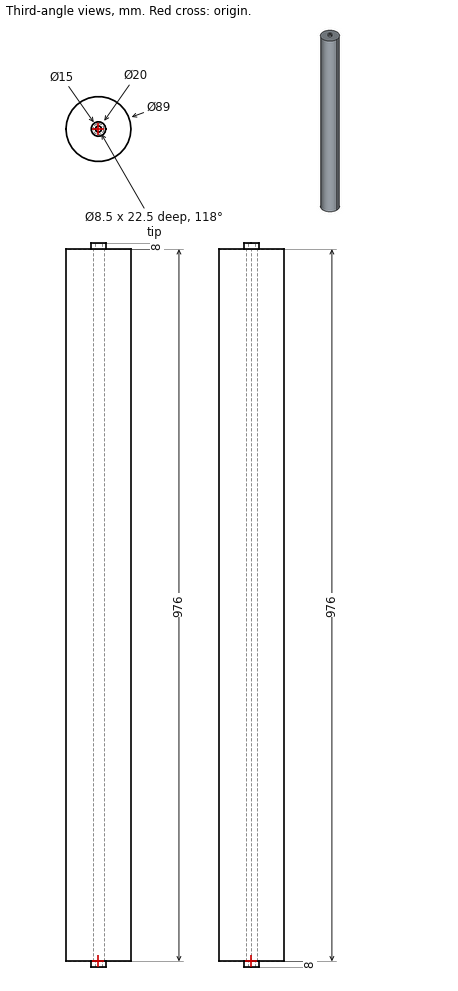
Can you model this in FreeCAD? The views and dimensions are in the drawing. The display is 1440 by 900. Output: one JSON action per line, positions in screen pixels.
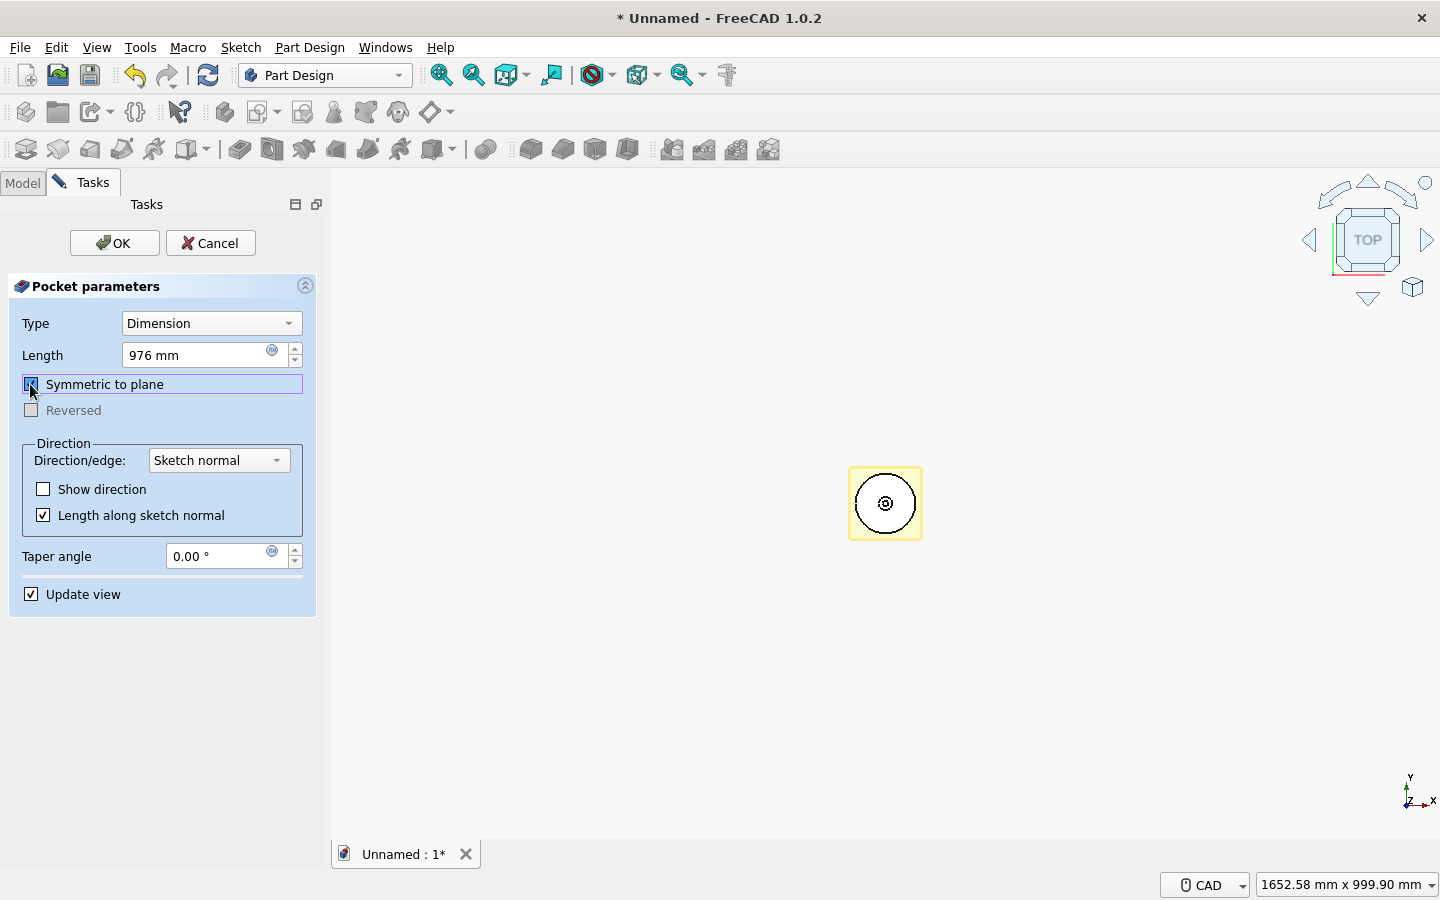
{"action": "left_click", "coordinate": [115, 243]}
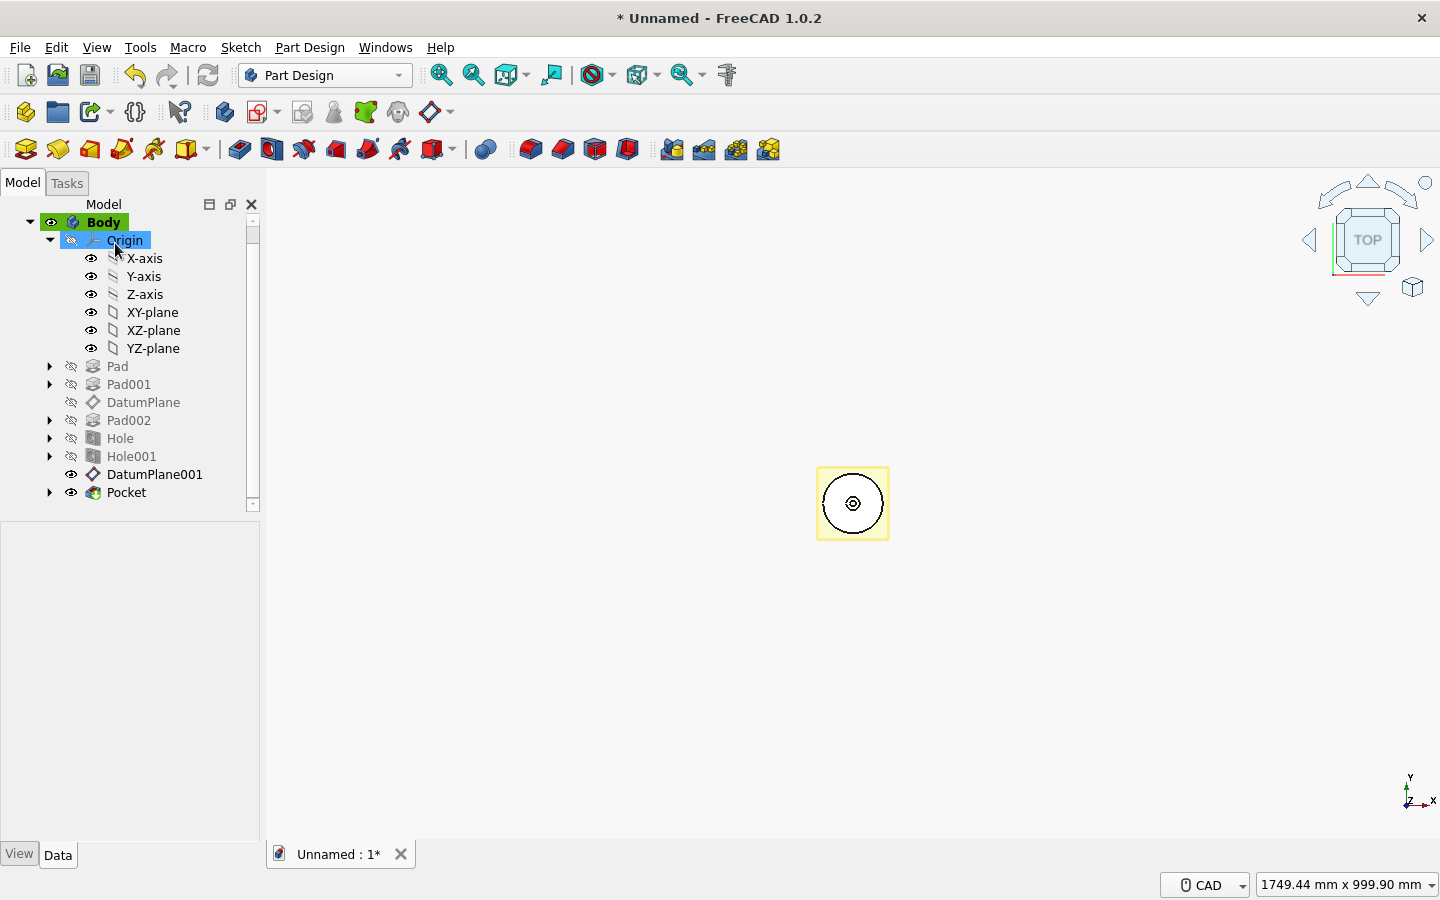
{"action": "left_click", "coordinate": [116, 474]}
{"action": "key", "text": "space"}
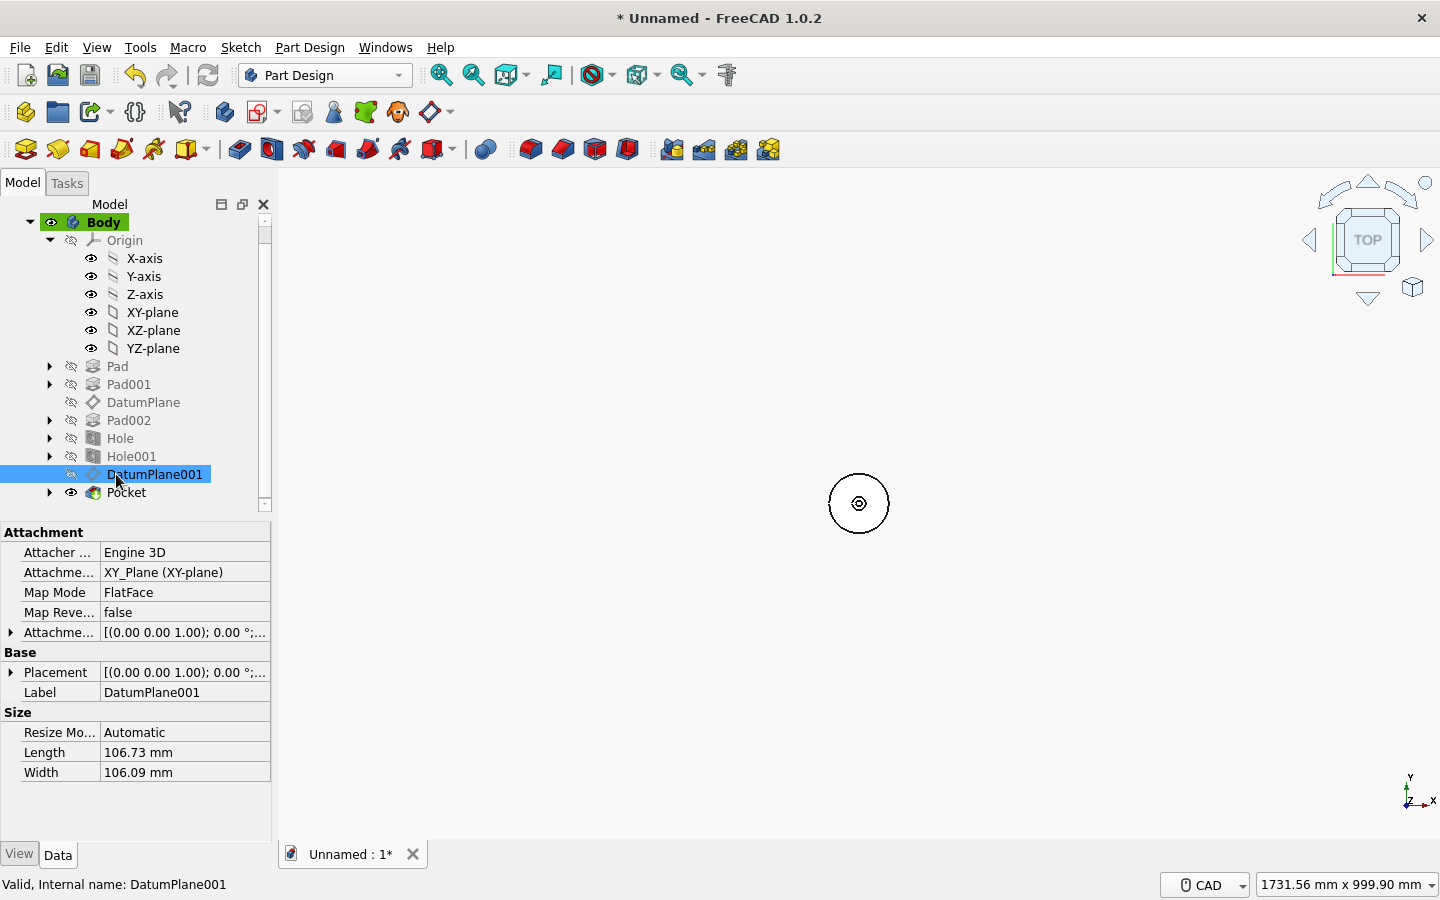
{"action": "key", "text": "0"}